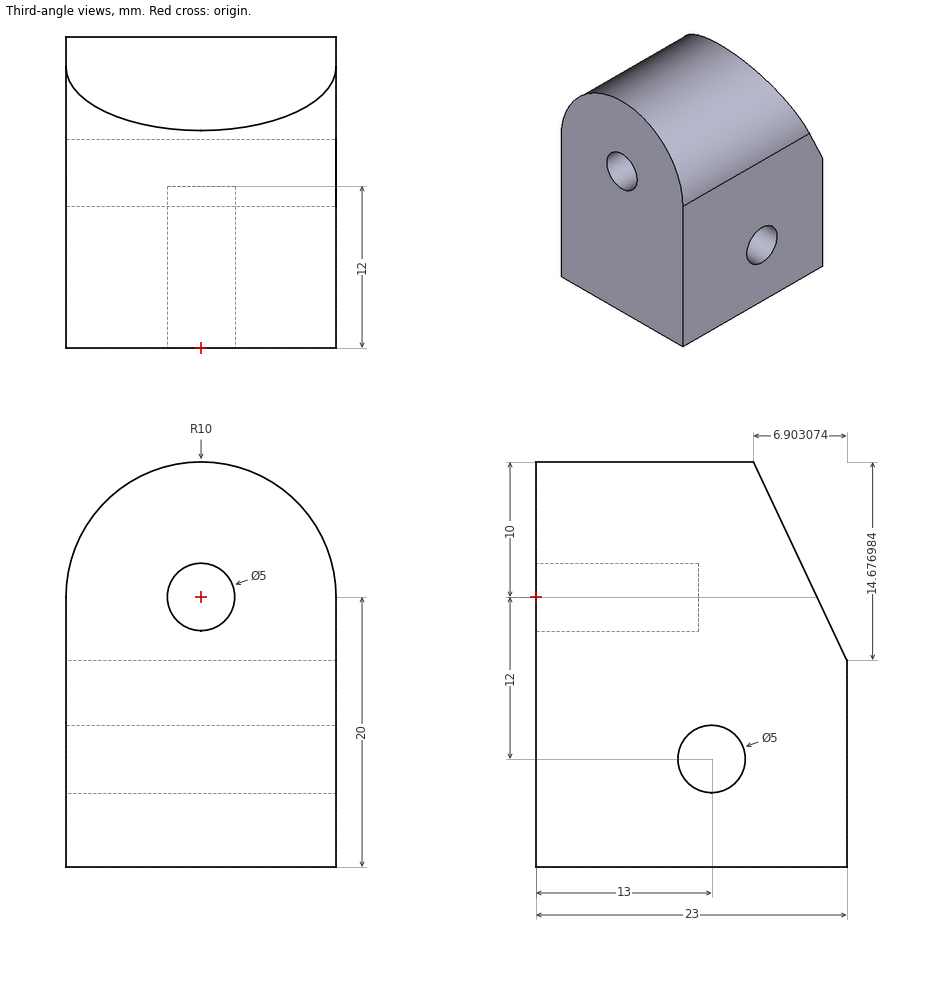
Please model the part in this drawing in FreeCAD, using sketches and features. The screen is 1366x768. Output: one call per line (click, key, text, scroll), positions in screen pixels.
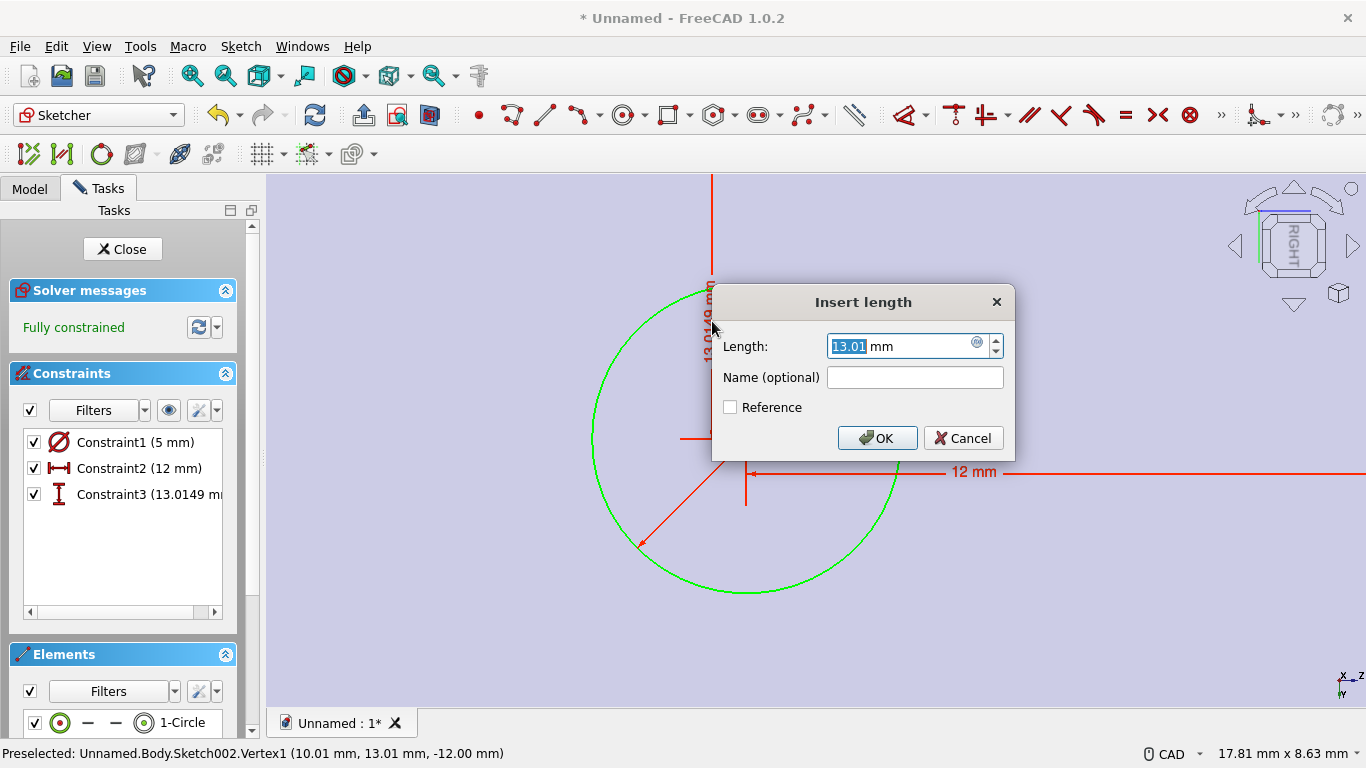
text(13)
key(Return)
key(Escape)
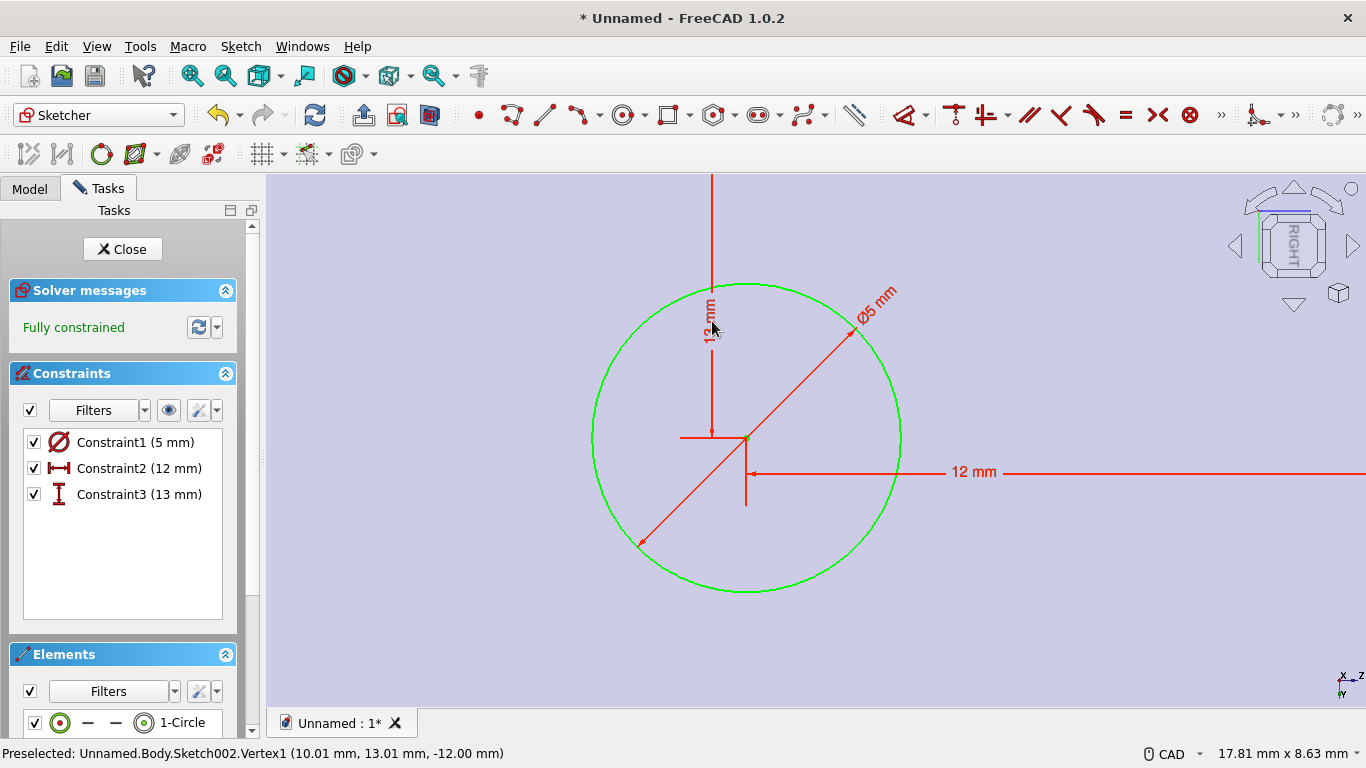
click(123, 249)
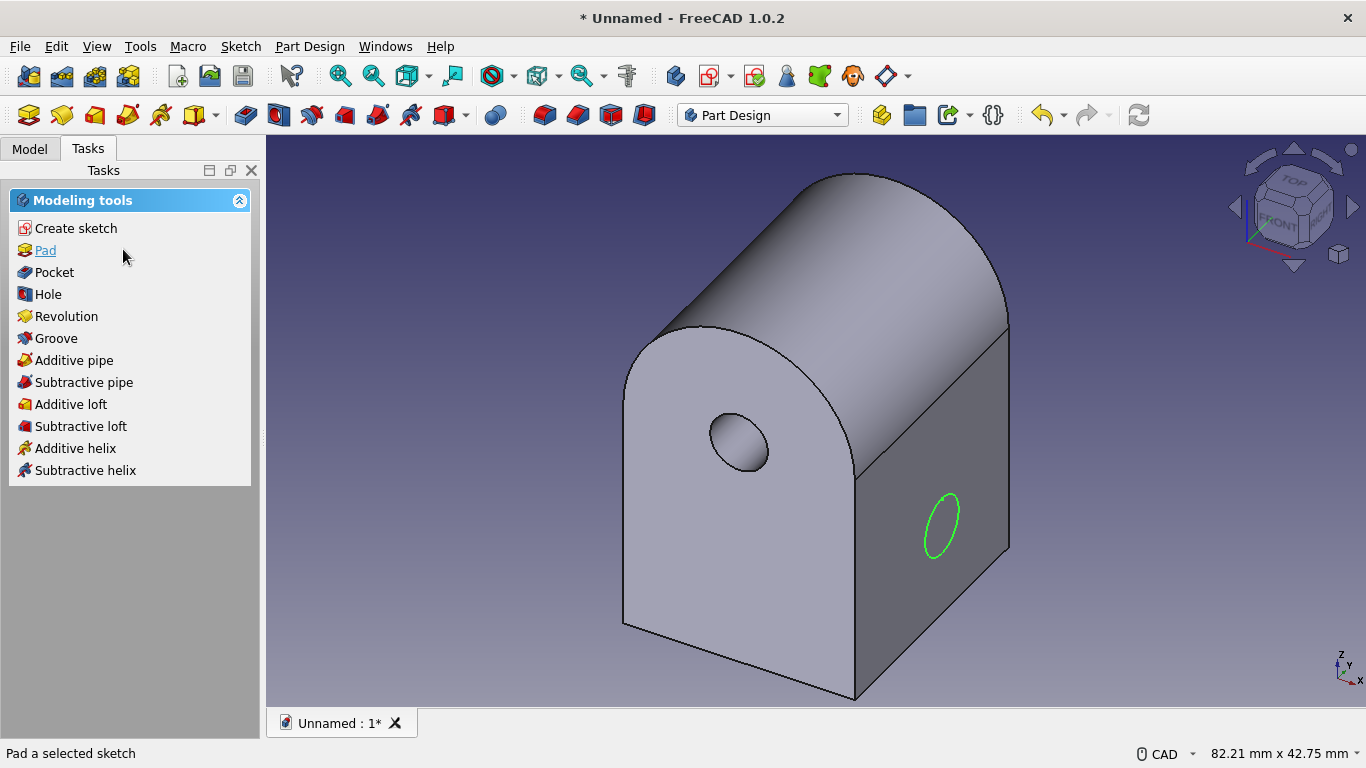
click(246, 116)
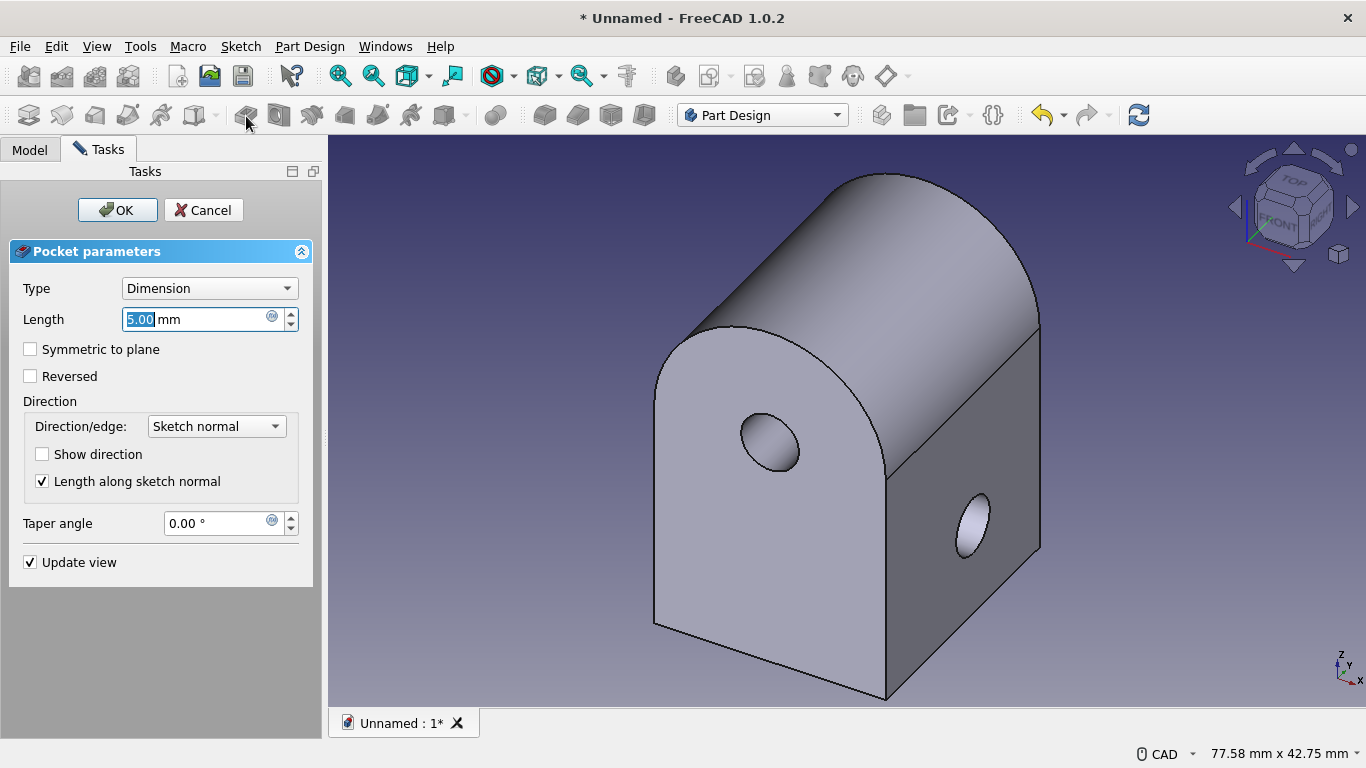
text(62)
key(Tab)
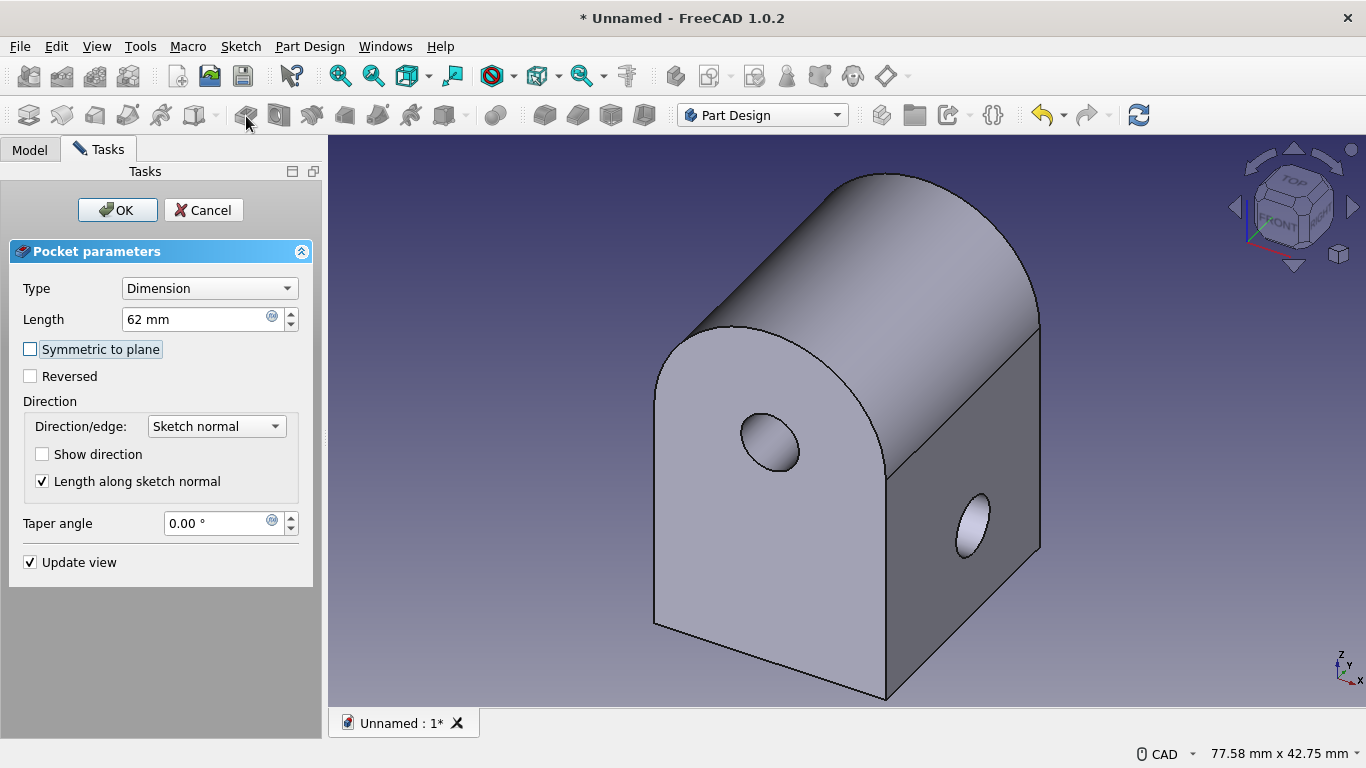
click(118, 210)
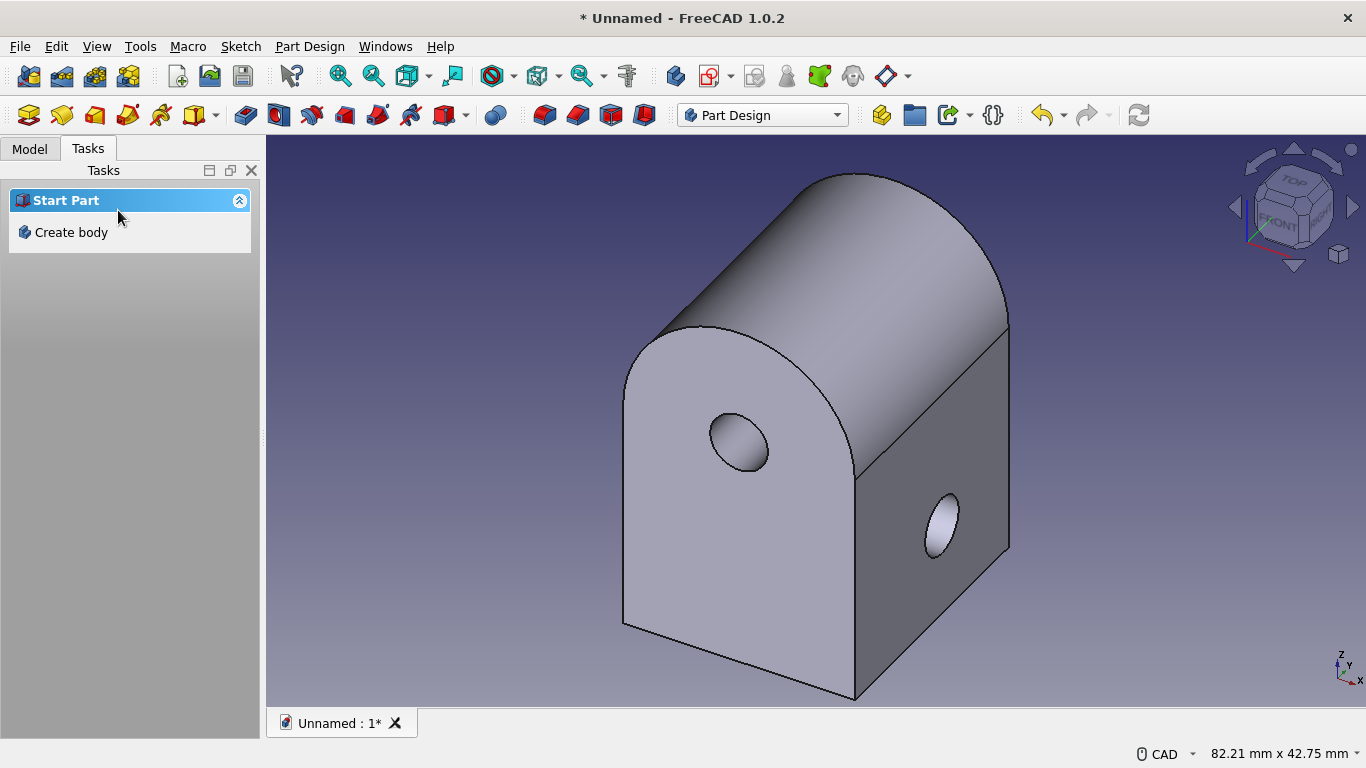
click(888, 525)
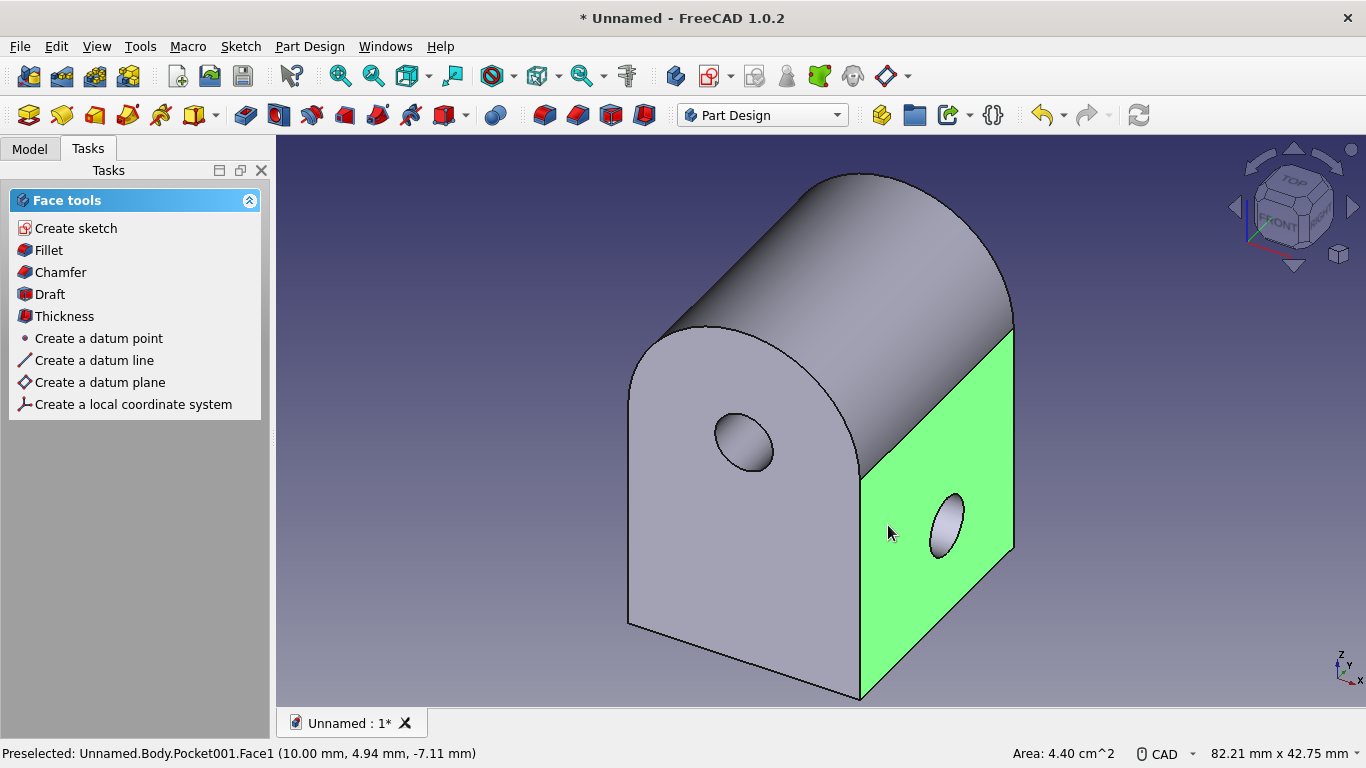
click(708, 76)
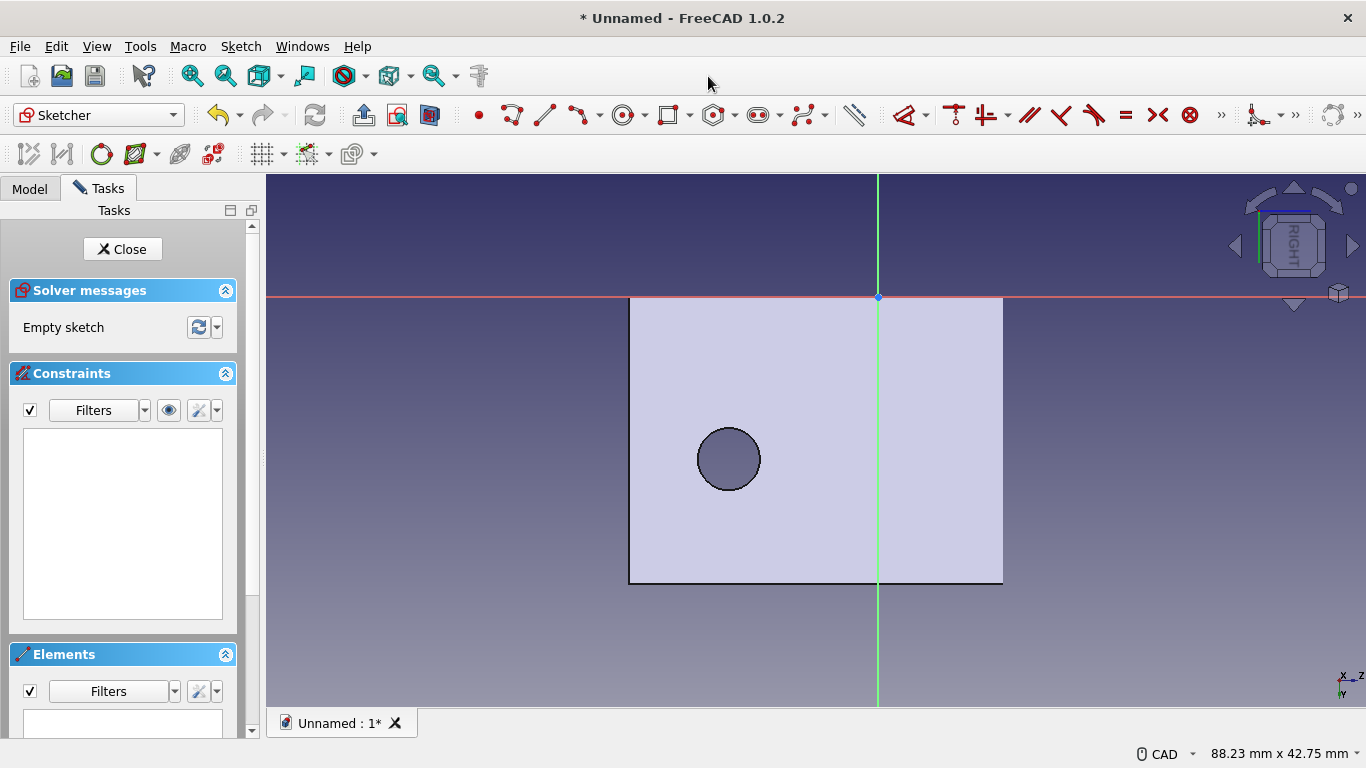
click(512, 116)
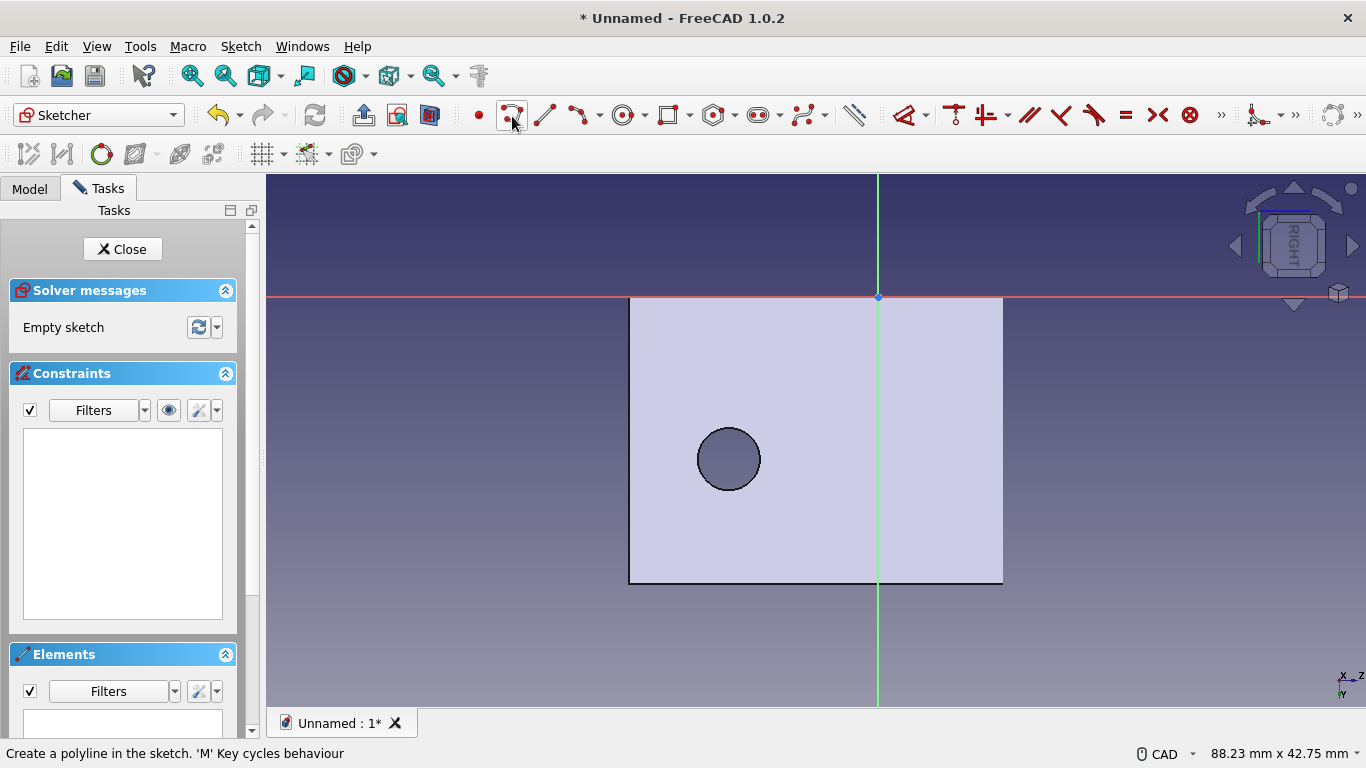
click(1003, 498)
click(820, 584)
click(1003, 584)
click(1003, 499)
key(Escape)
key(Escape)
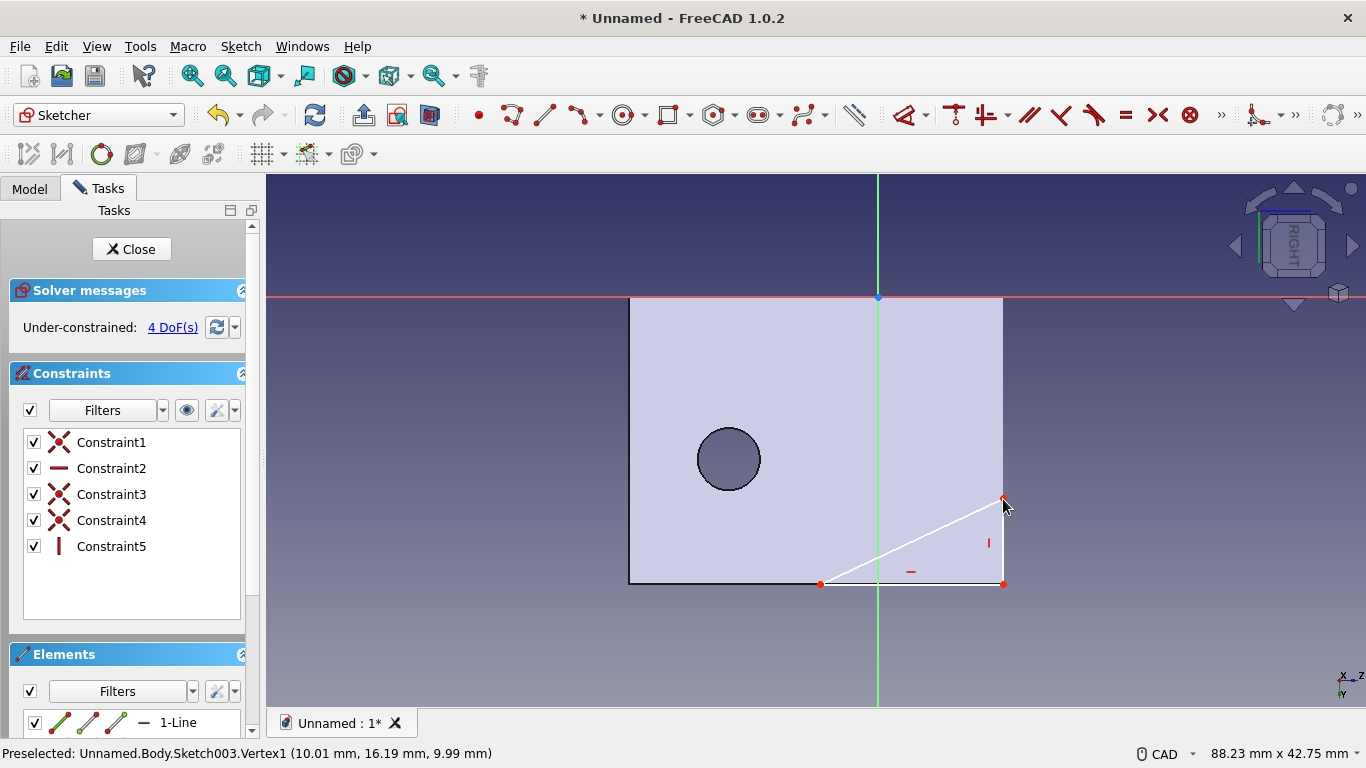
key(d)